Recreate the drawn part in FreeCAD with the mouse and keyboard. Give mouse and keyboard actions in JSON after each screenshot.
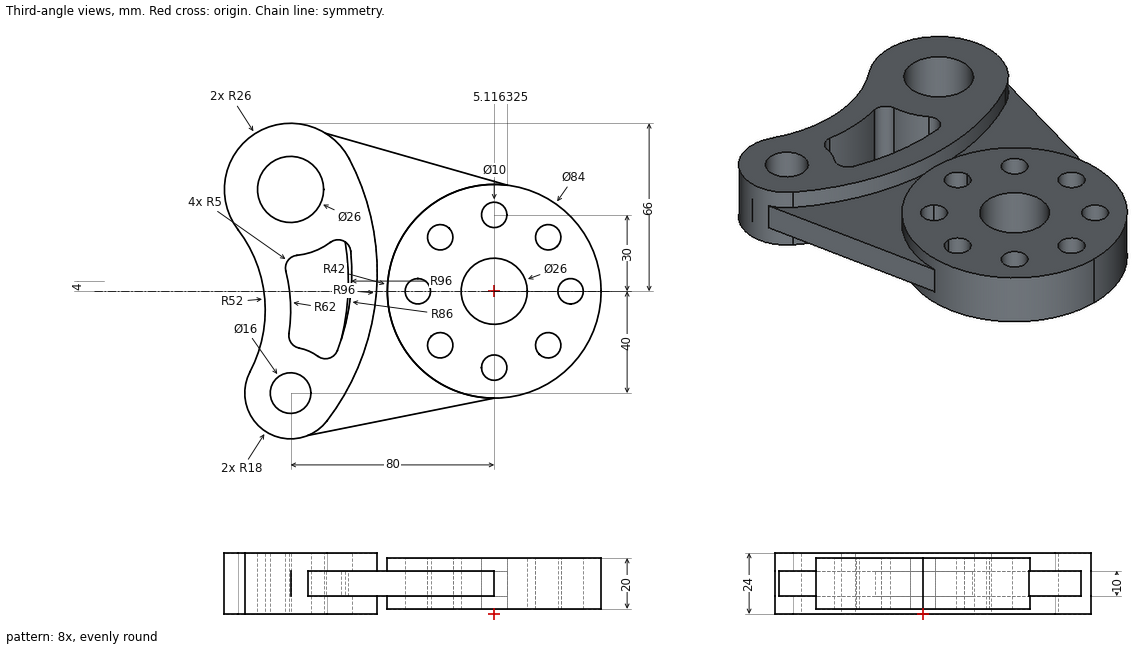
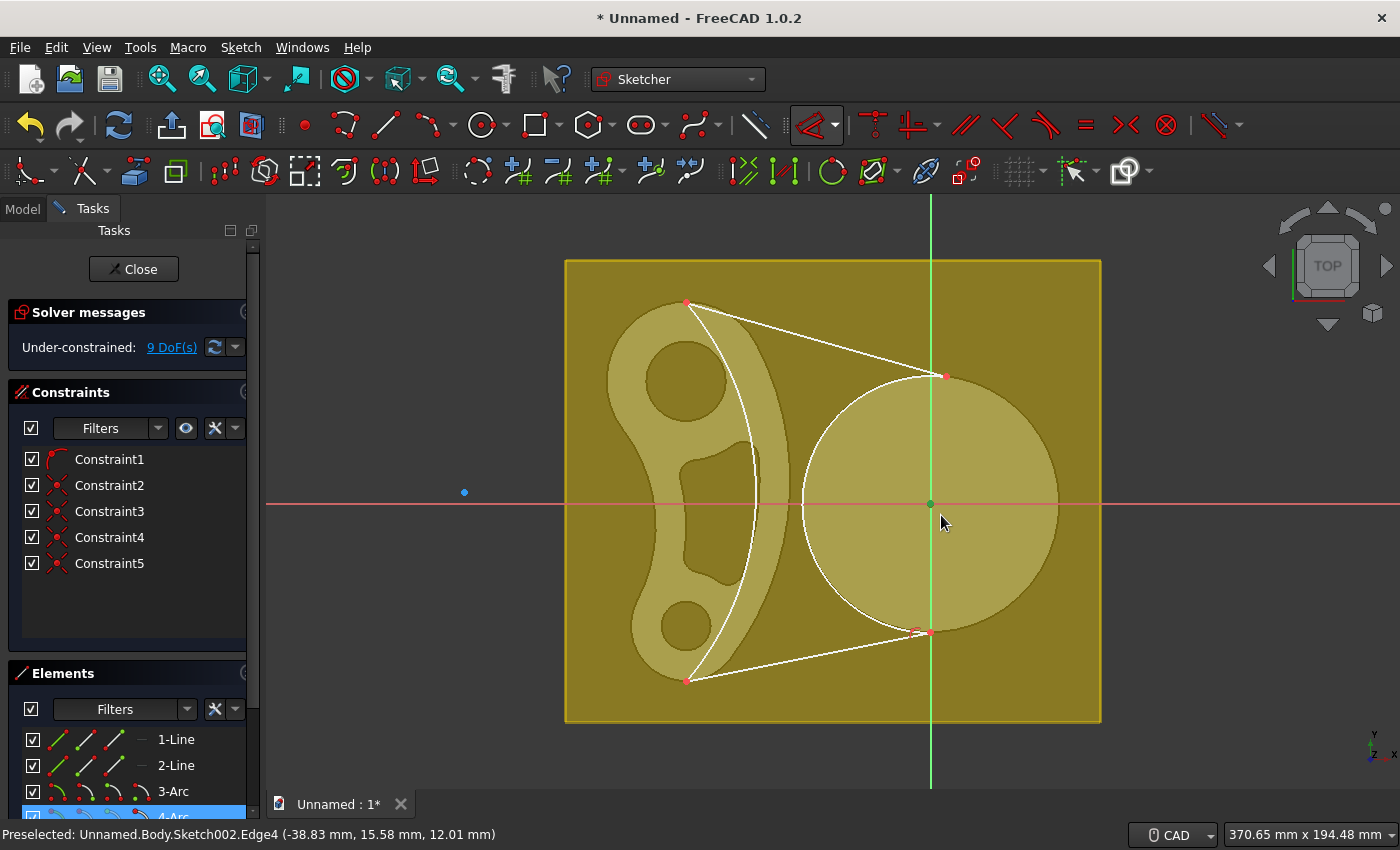
{"action": "left_click", "coordinate": [874, 126]}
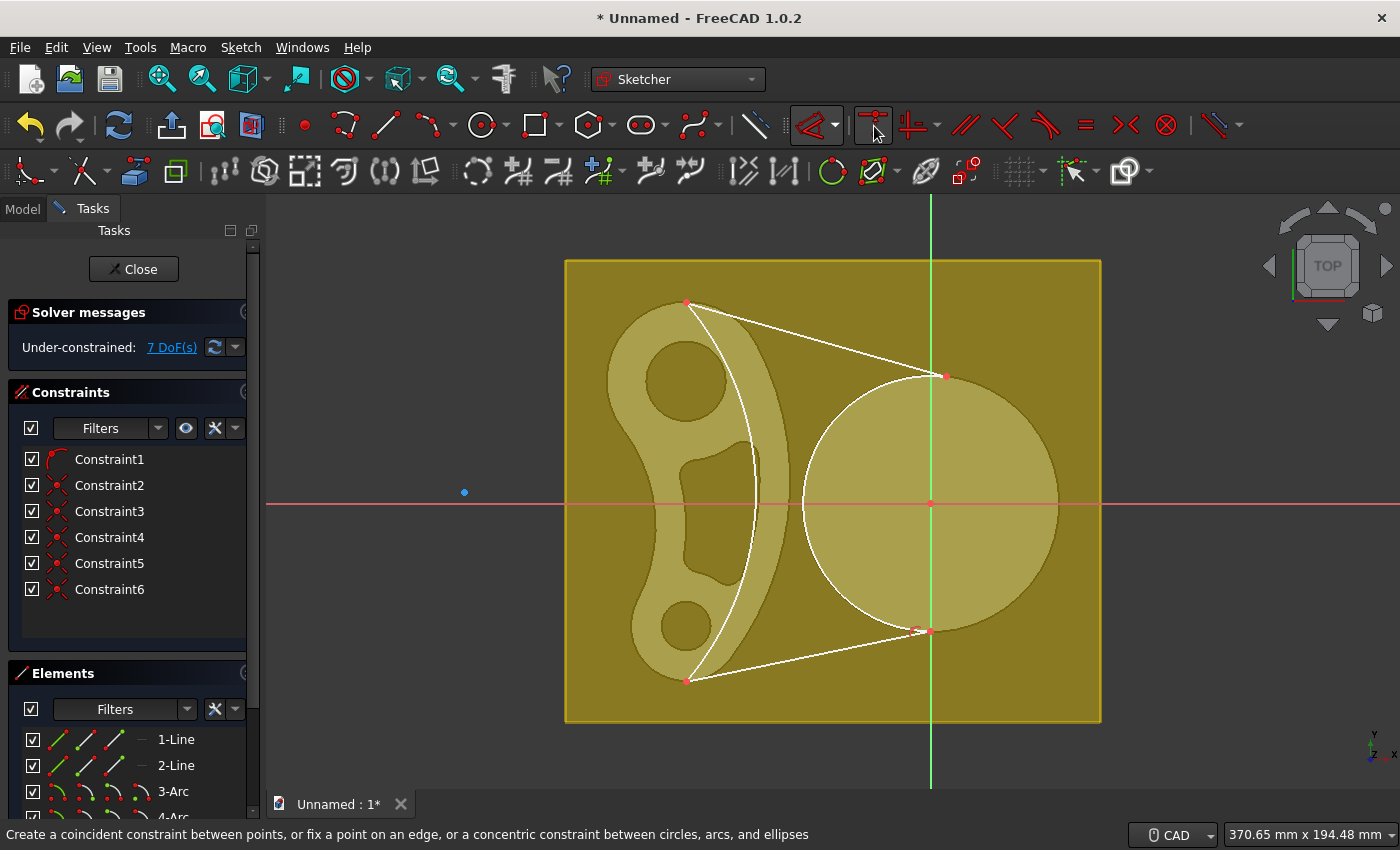
{"action": "left_click", "coordinate": [744, 574]}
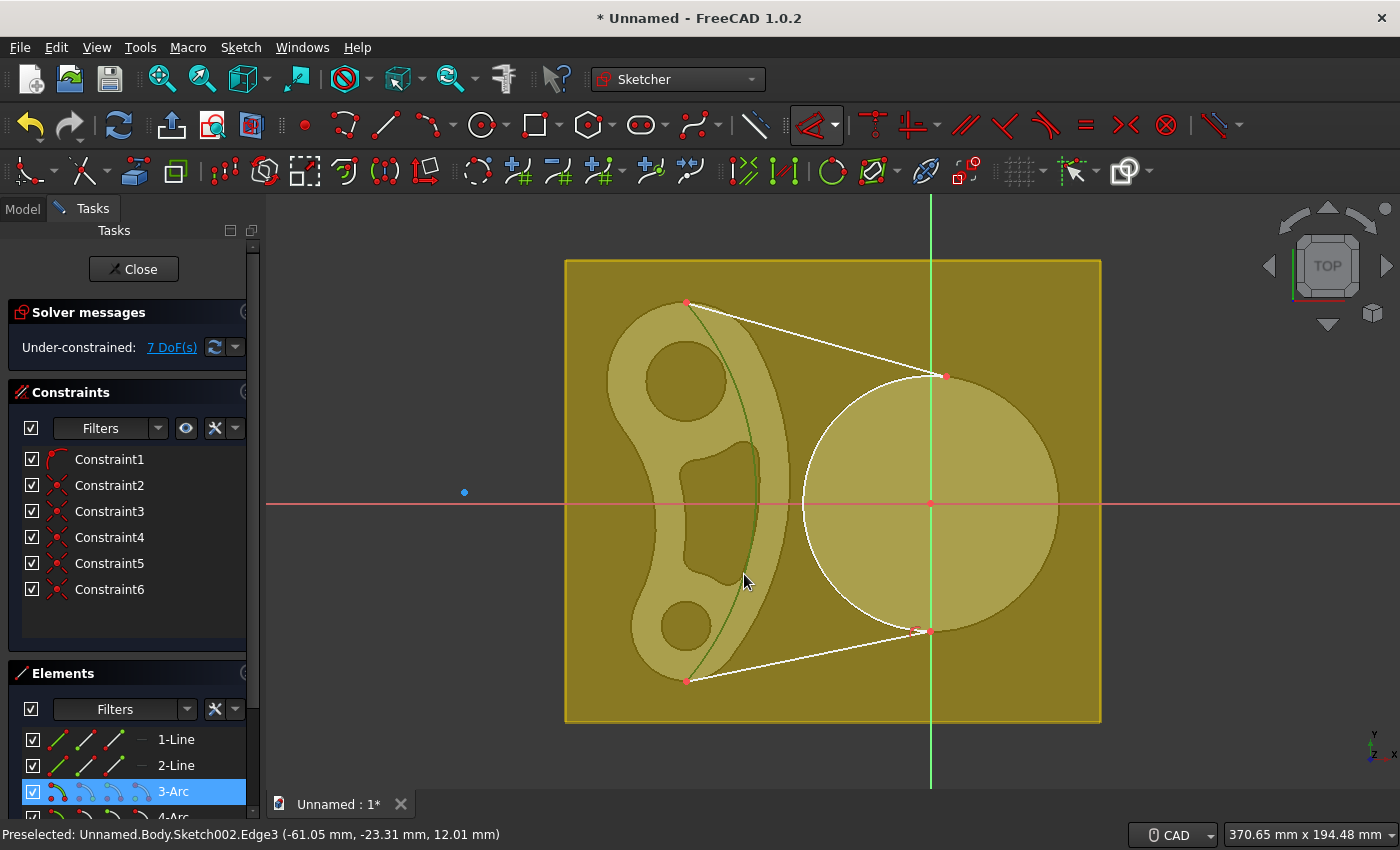
{"action": "left_click", "coordinate": [838, 126]}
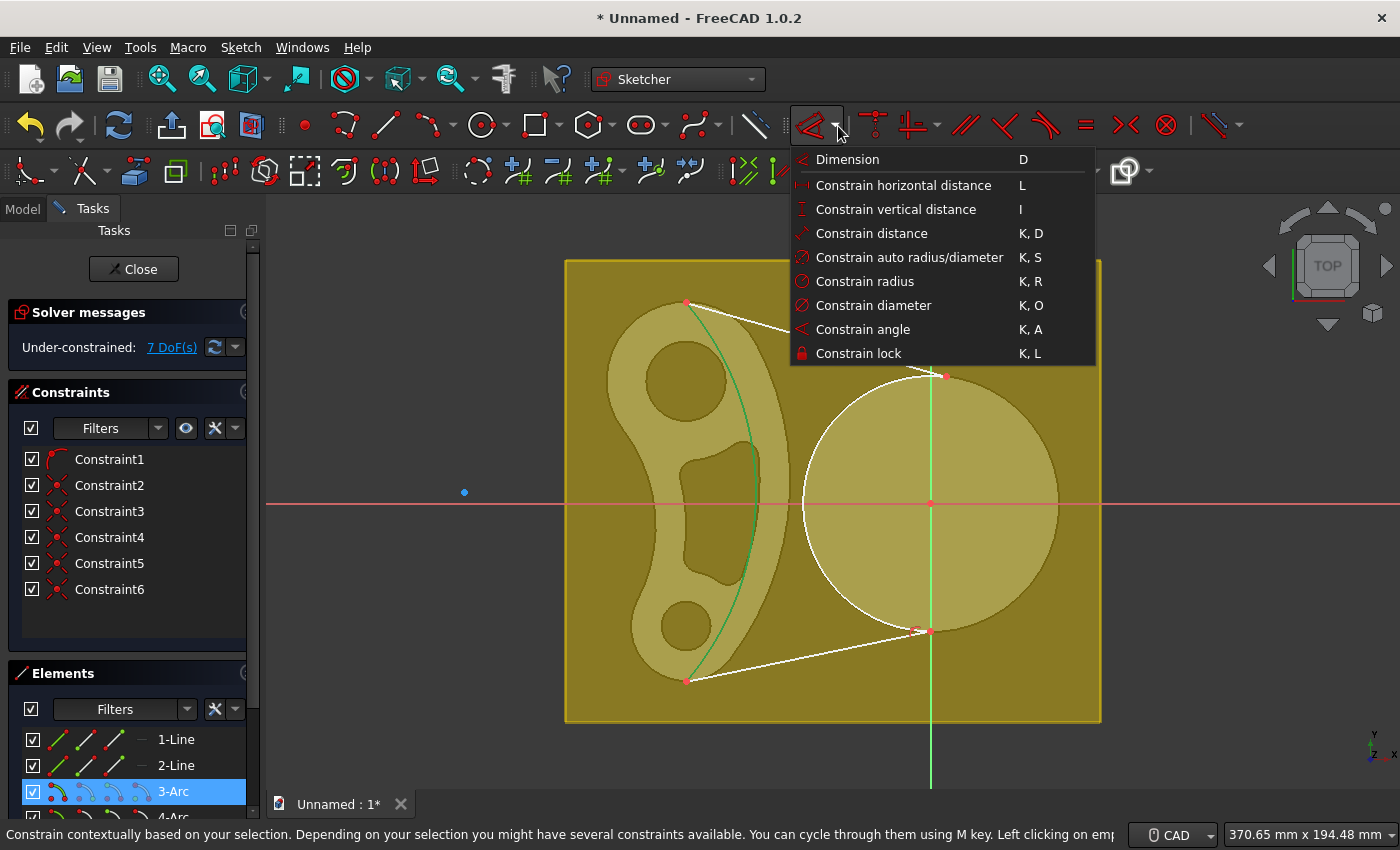
{"action": "left_click", "coordinate": [943, 281]}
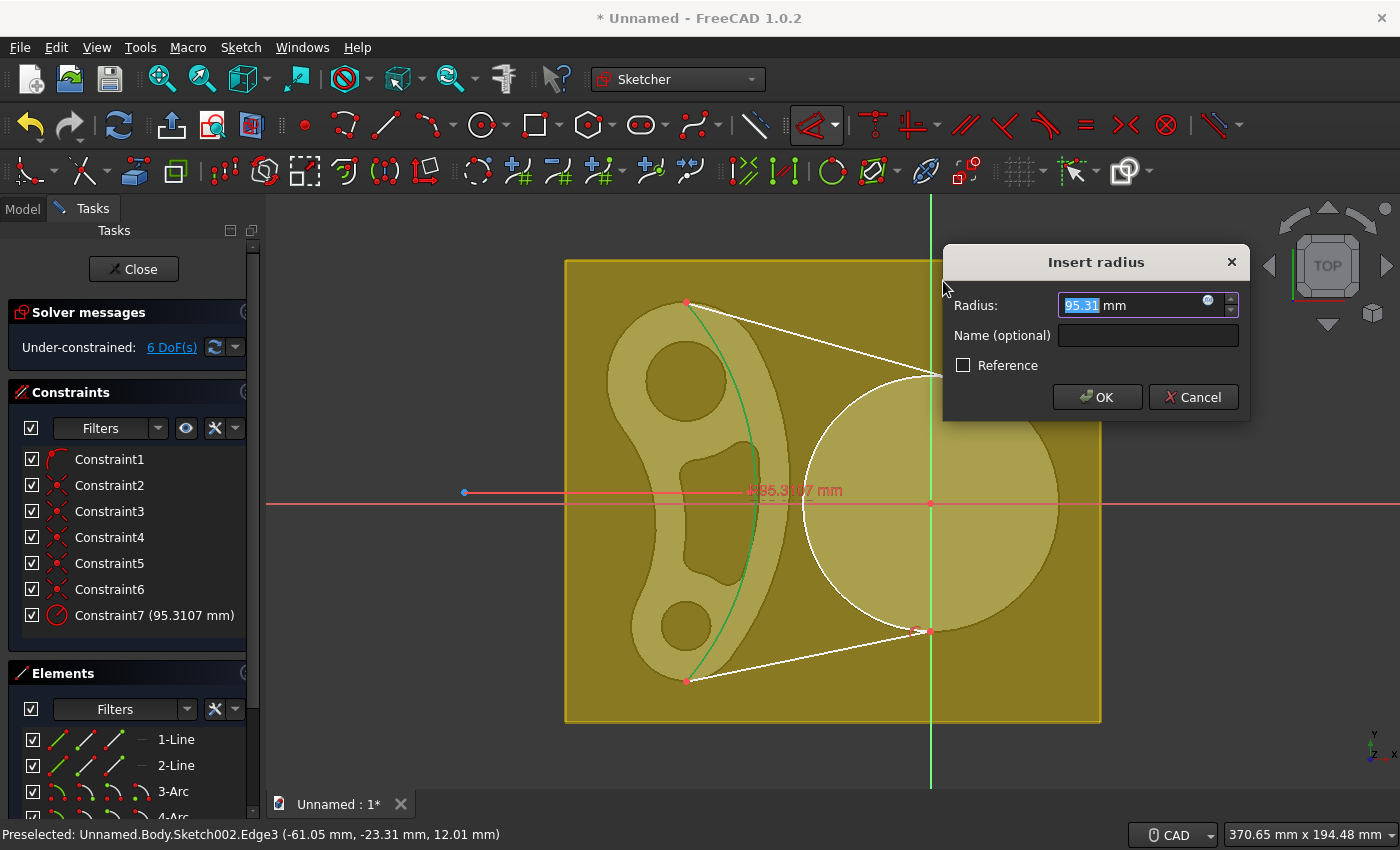
{"action": "type", "text": "96"}
{"action": "key", "text": "Return"}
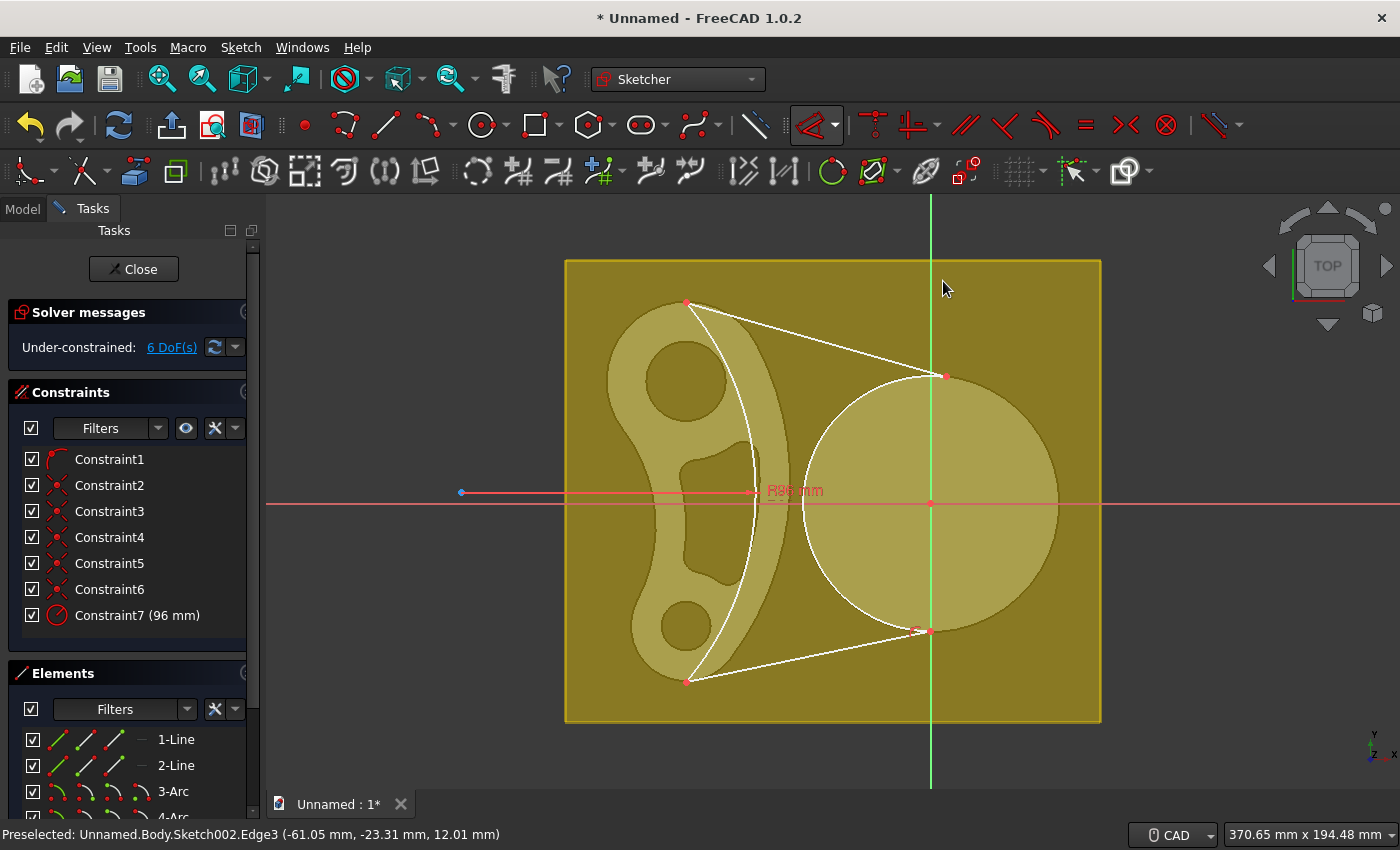
{"action": "left_click", "coordinate": [834, 420]}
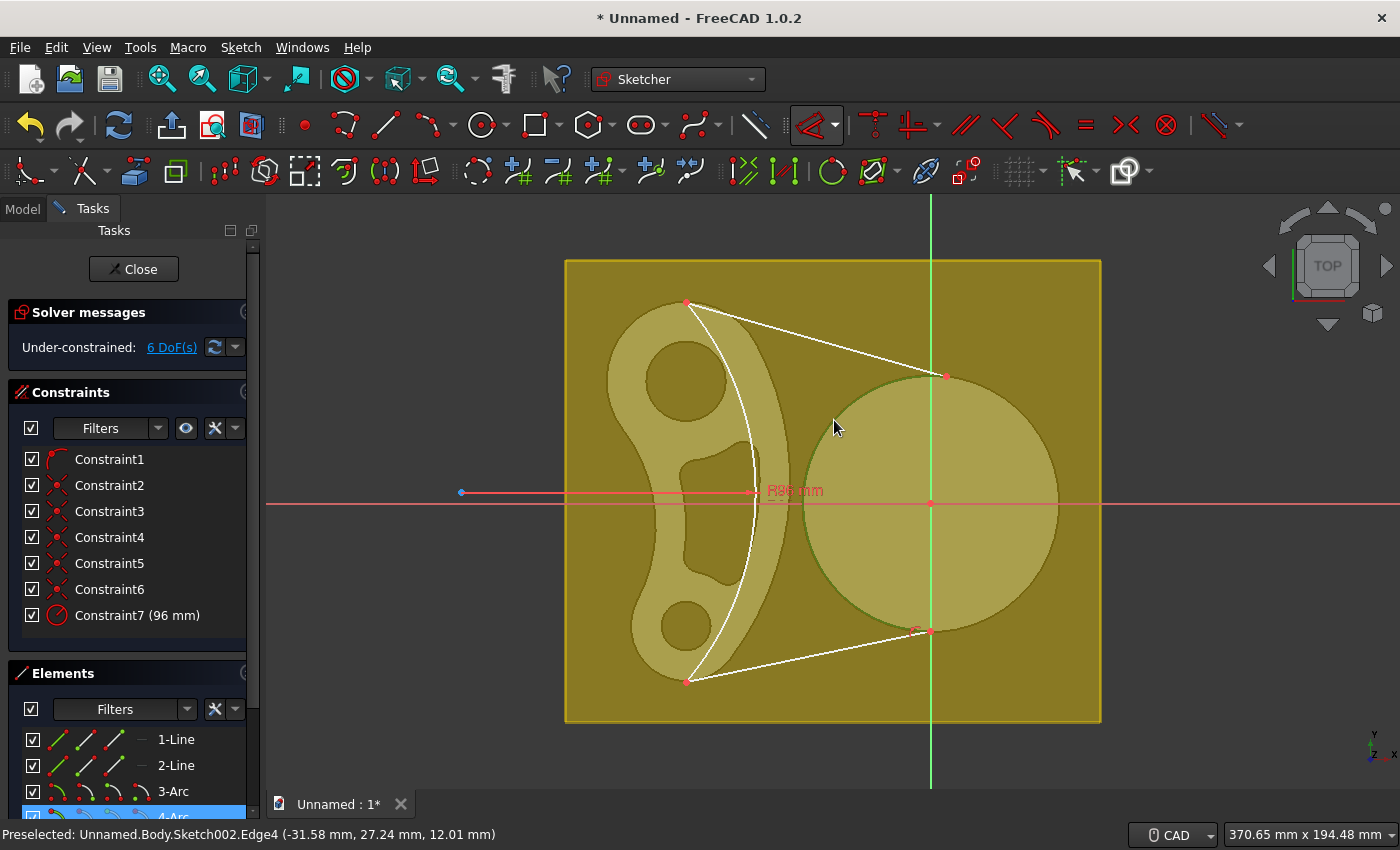
{"action": "key", "text": "k r"}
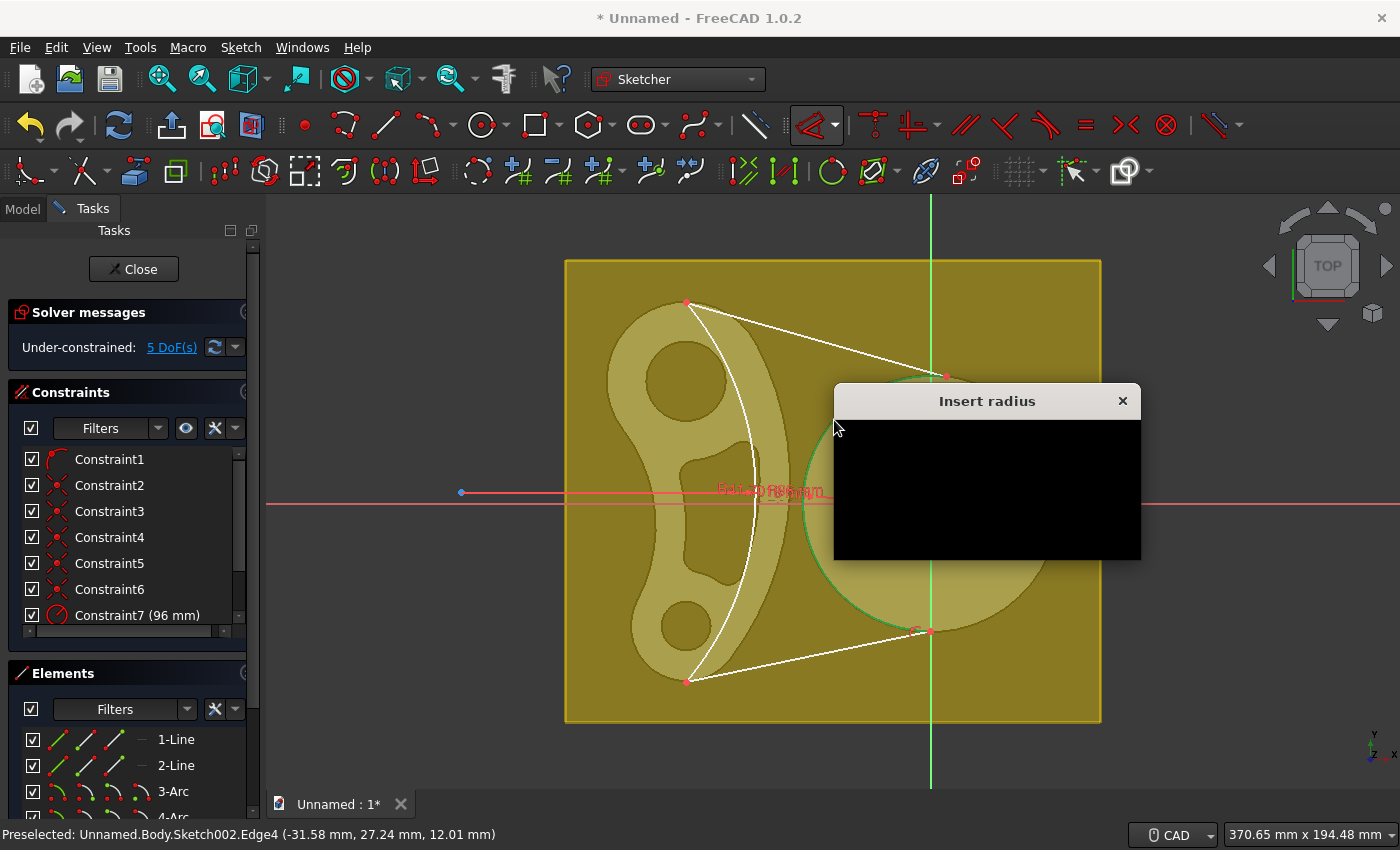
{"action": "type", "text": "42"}
{"action": "key", "text": "Return"}